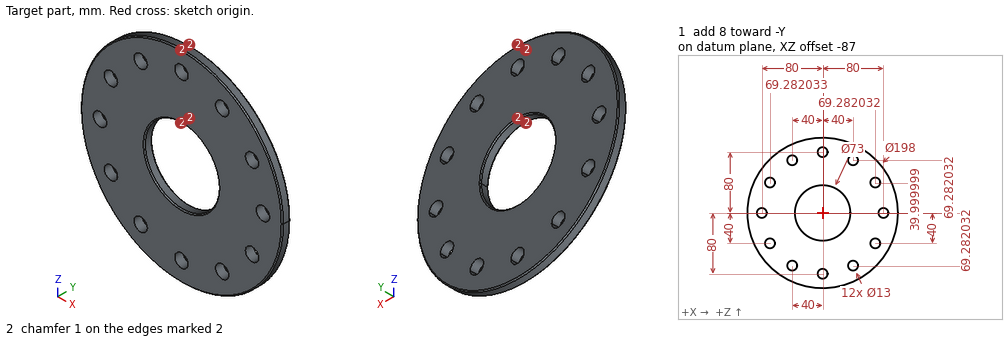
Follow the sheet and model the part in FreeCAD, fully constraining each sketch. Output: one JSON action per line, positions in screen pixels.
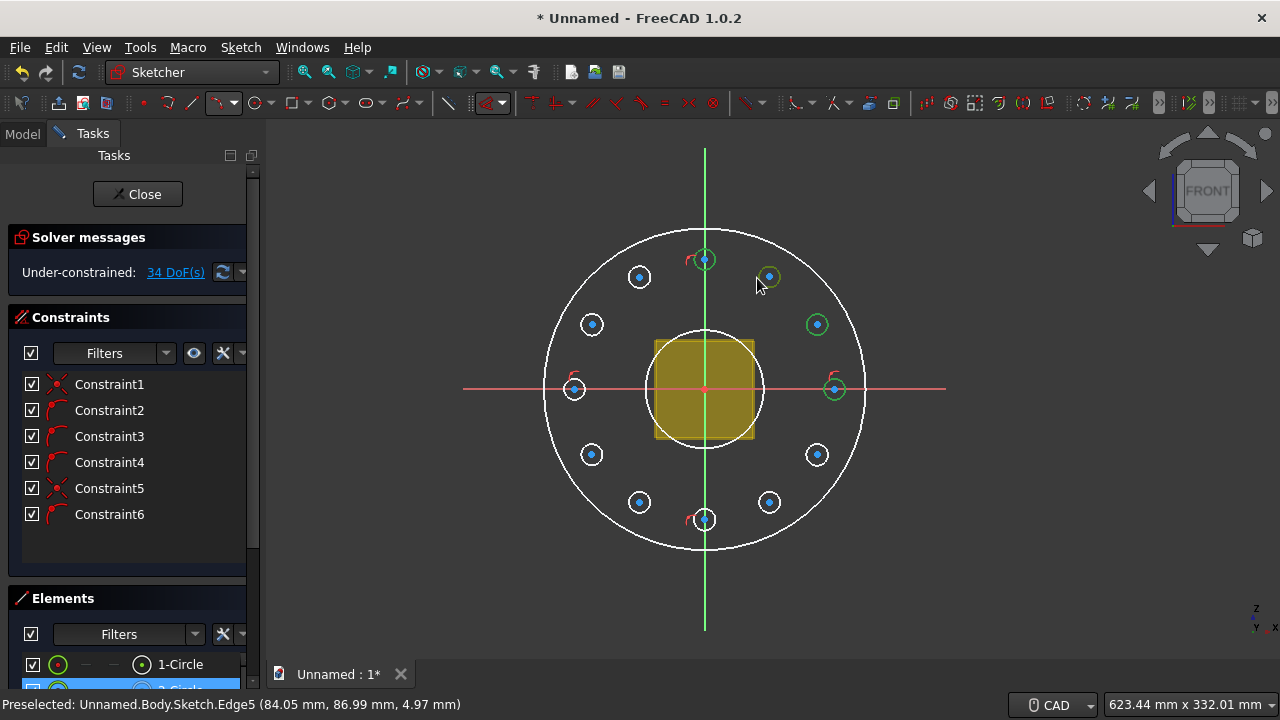
{"action": "scroll", "coordinate": [825, 447], "scroll_direction": "up", "scroll_amount": 2}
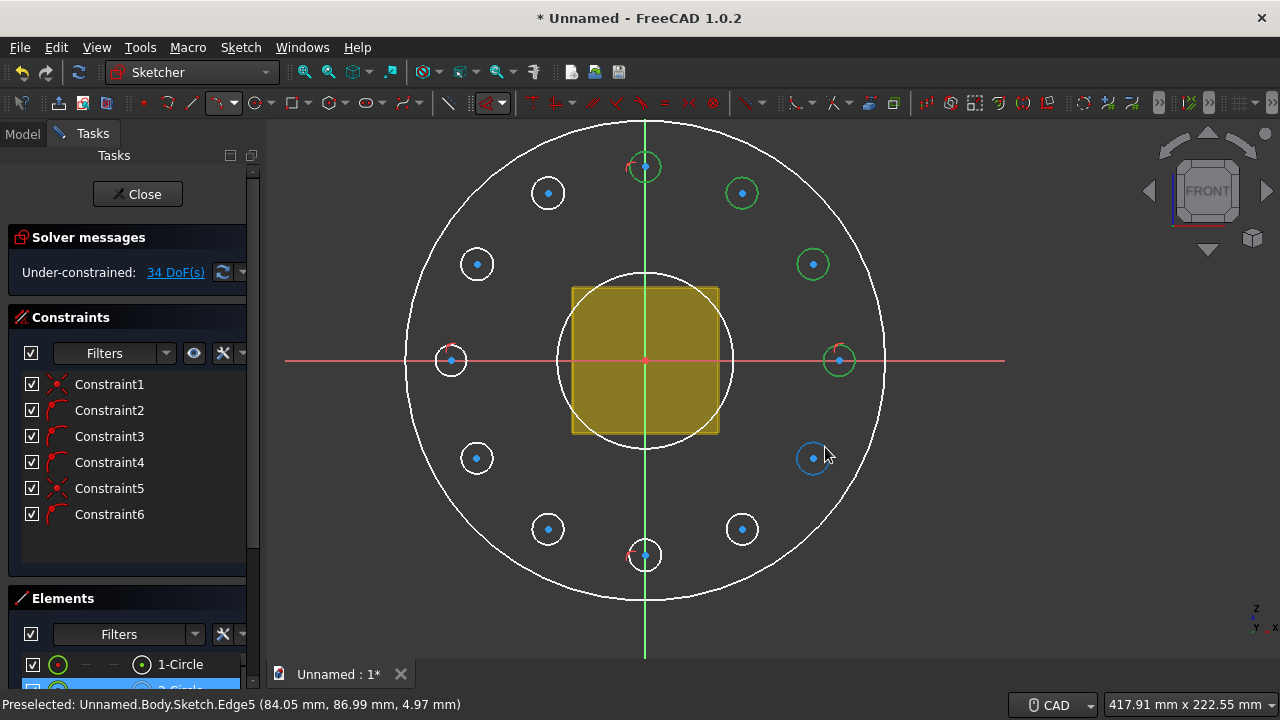
{"action": "left_click", "coordinate": [824, 447]}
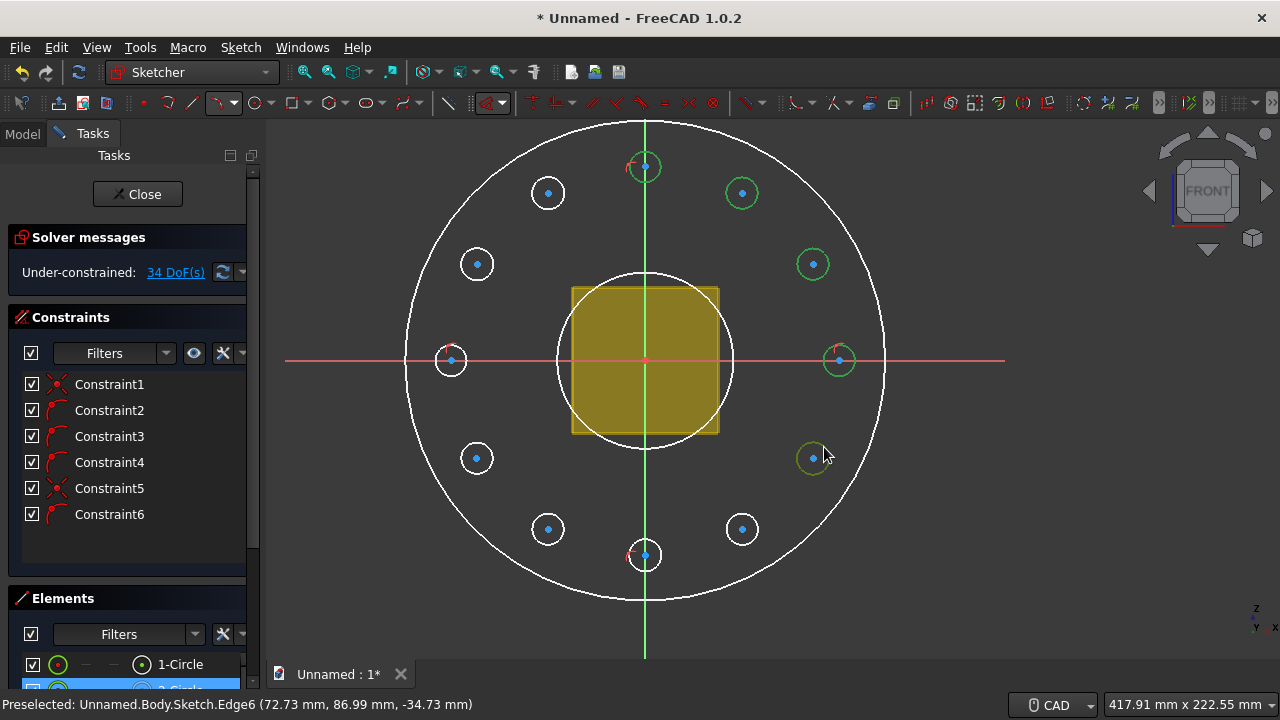
{"action": "left_click", "coordinate": [753, 518]}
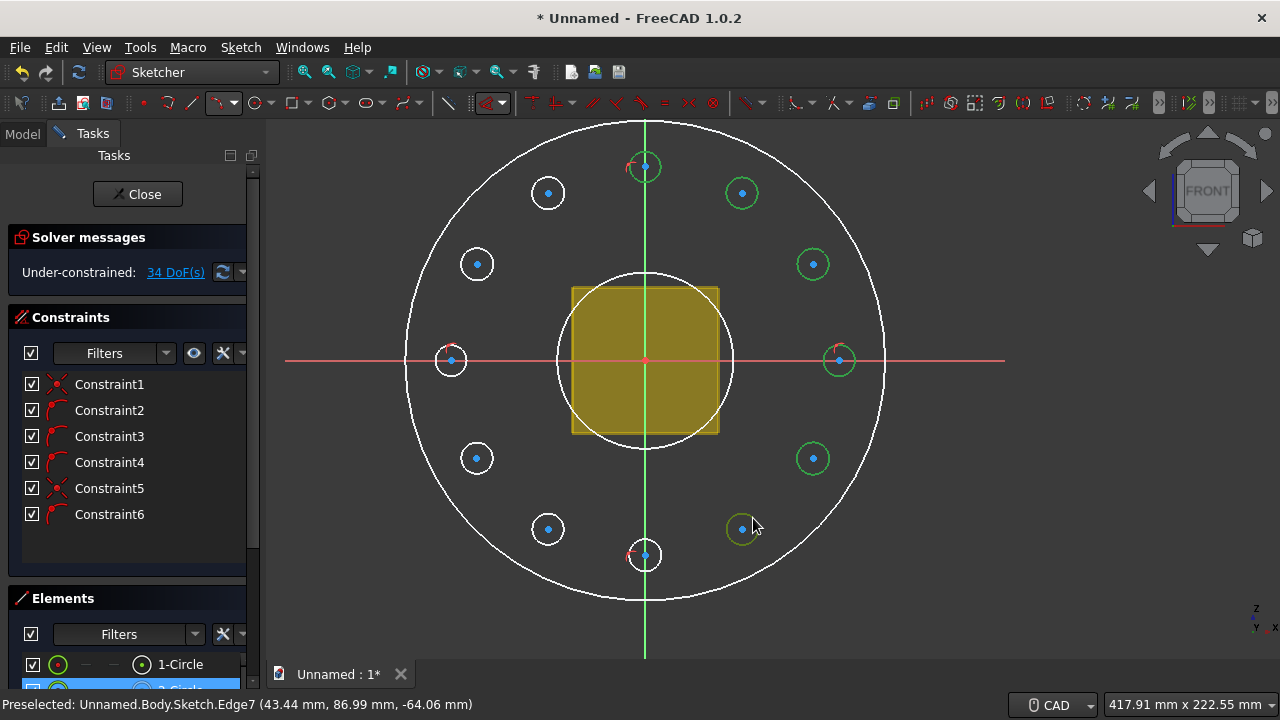
{"action": "left_click", "coordinate": [560, 182]}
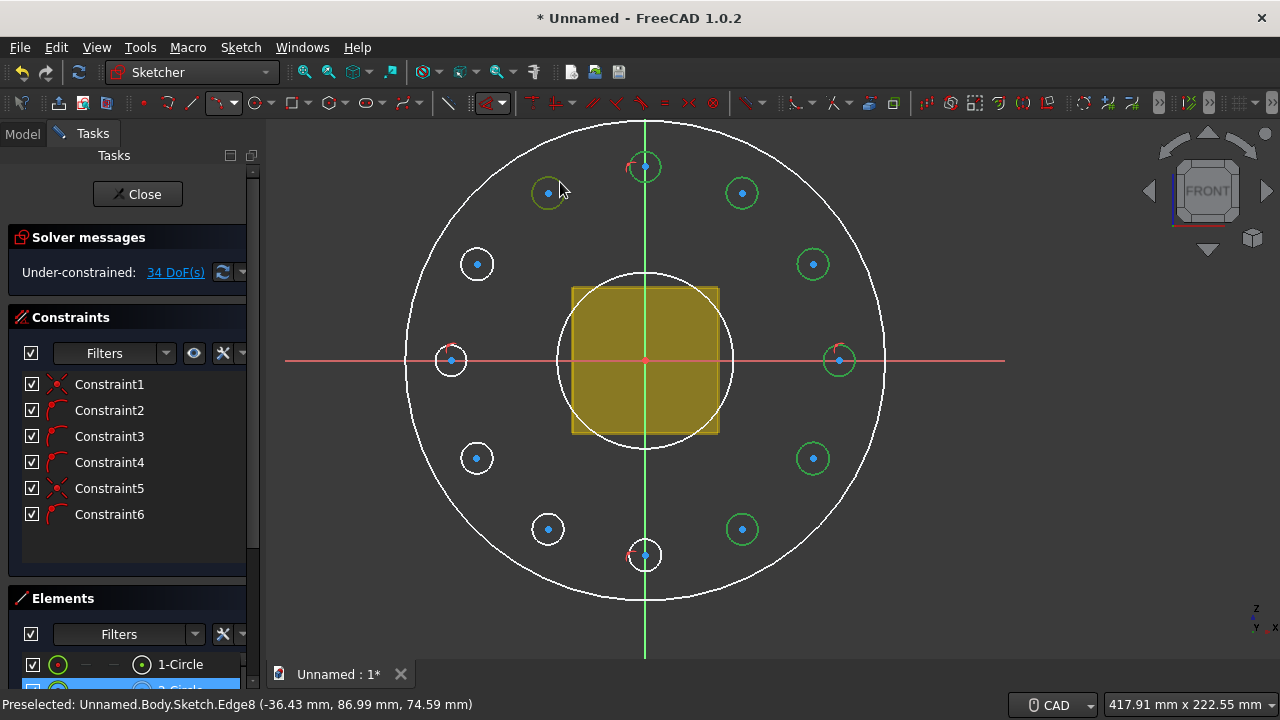
{"action": "left_click", "coordinate": [489, 253]}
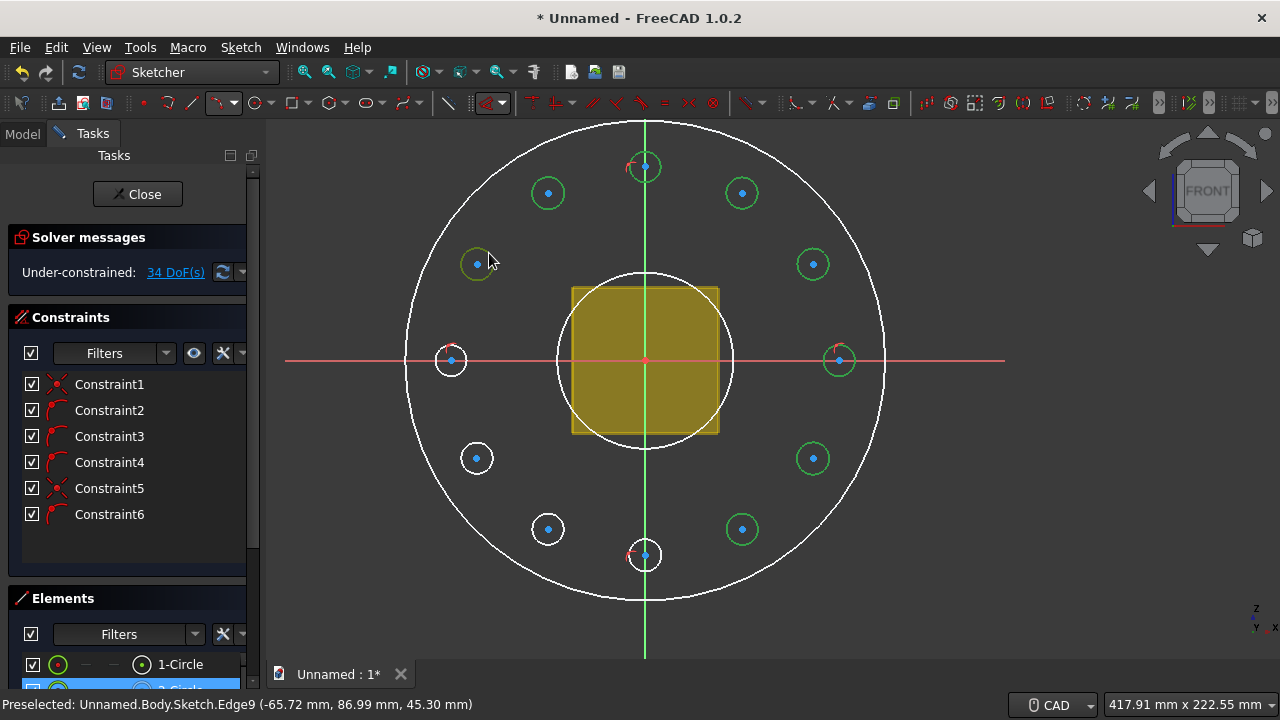
{"action": "scroll", "coordinate": [462, 350], "scroll_direction": "up", "scroll_amount": 2}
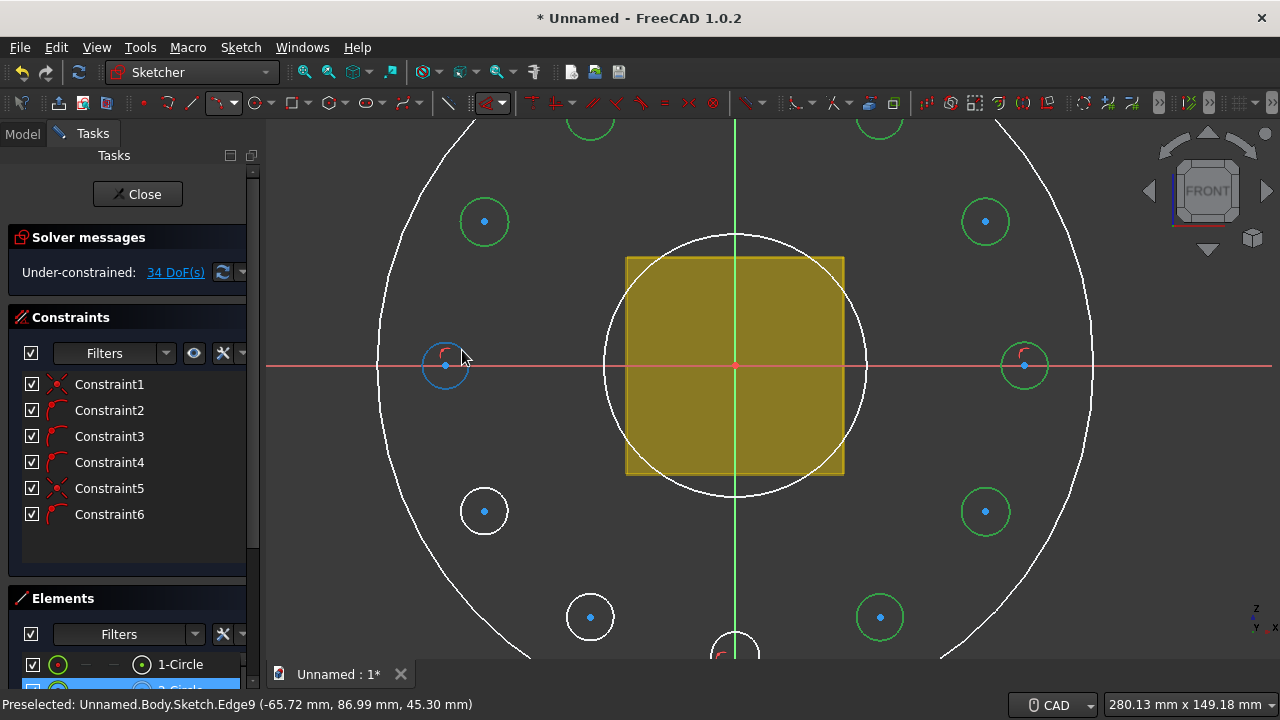
{"action": "left_click", "coordinate": [462, 349]}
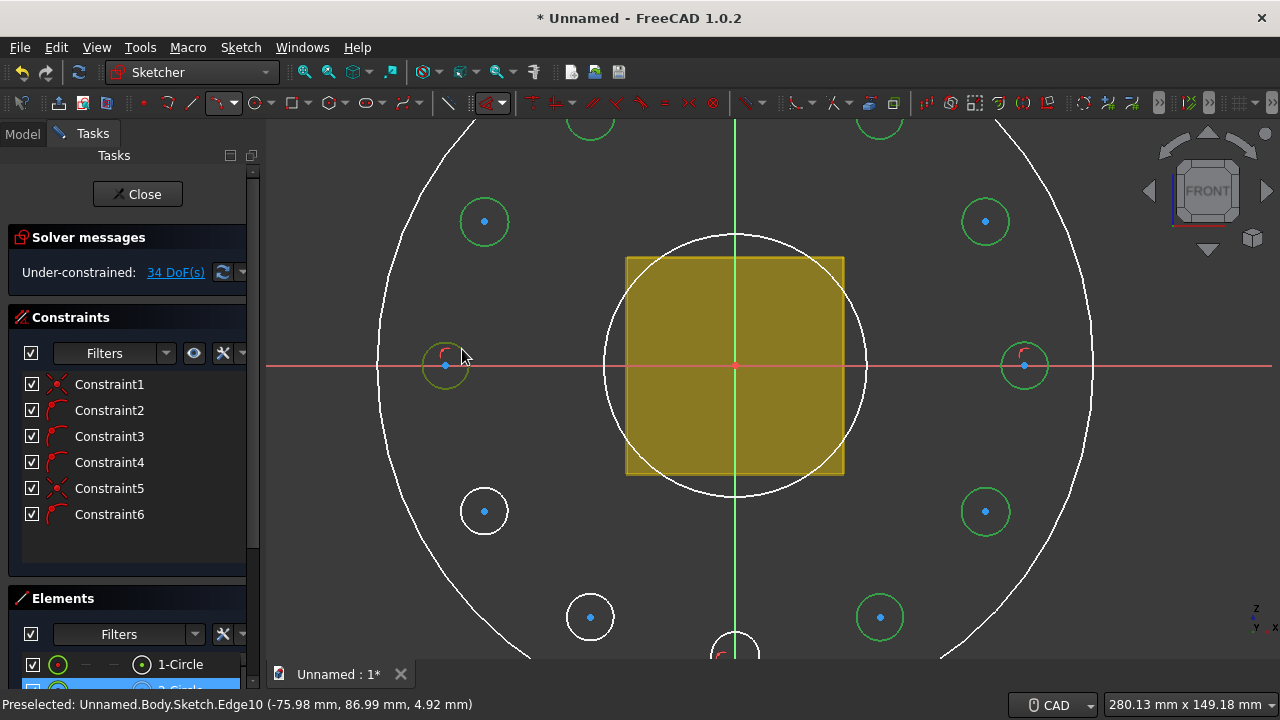
{"action": "scroll", "coordinate": [679, 408], "scroll_direction": "down", "scroll_amount": 4}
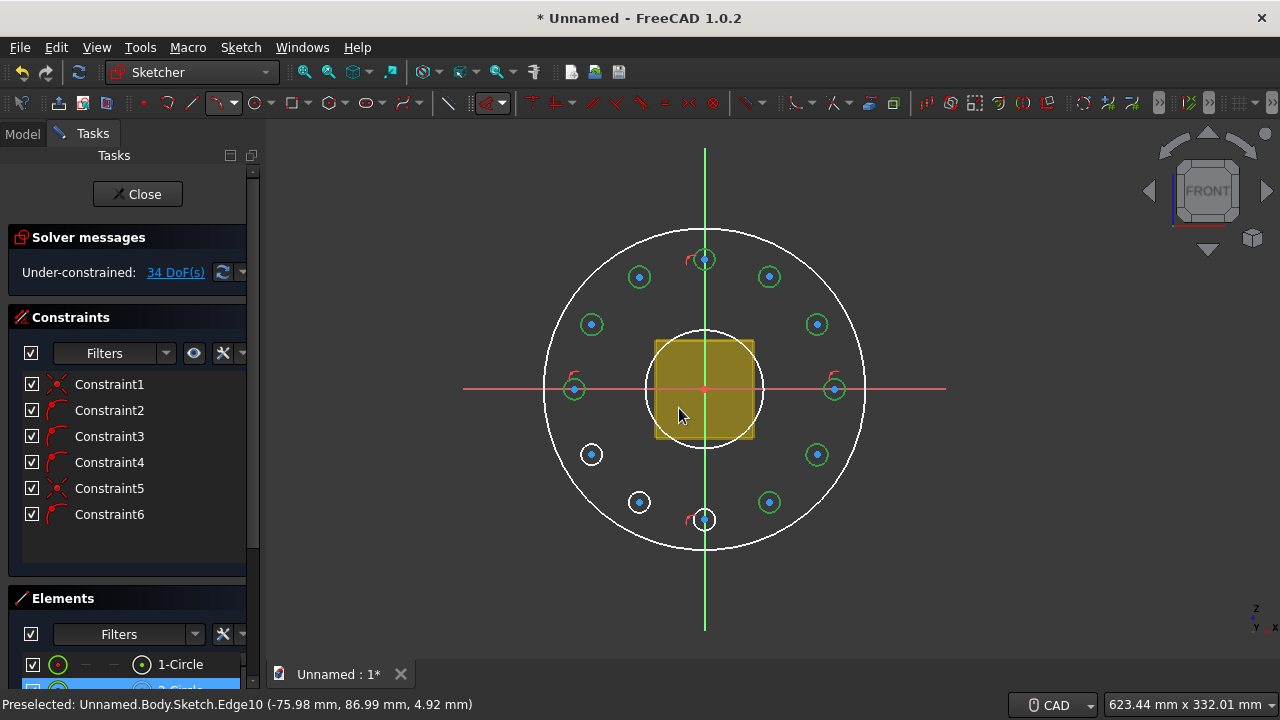
{"action": "scroll", "coordinate": [712, 512], "scroll_direction": "up", "scroll_amount": 3}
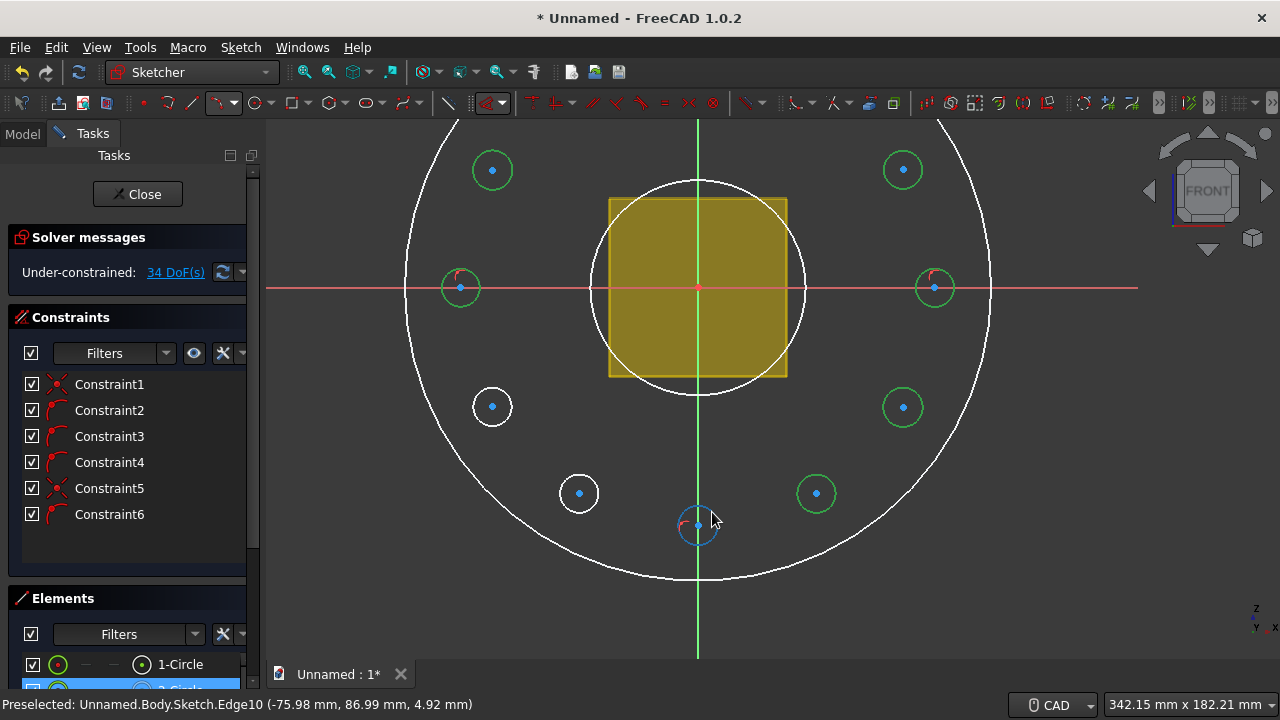
{"action": "left_click", "coordinate": [712, 512]}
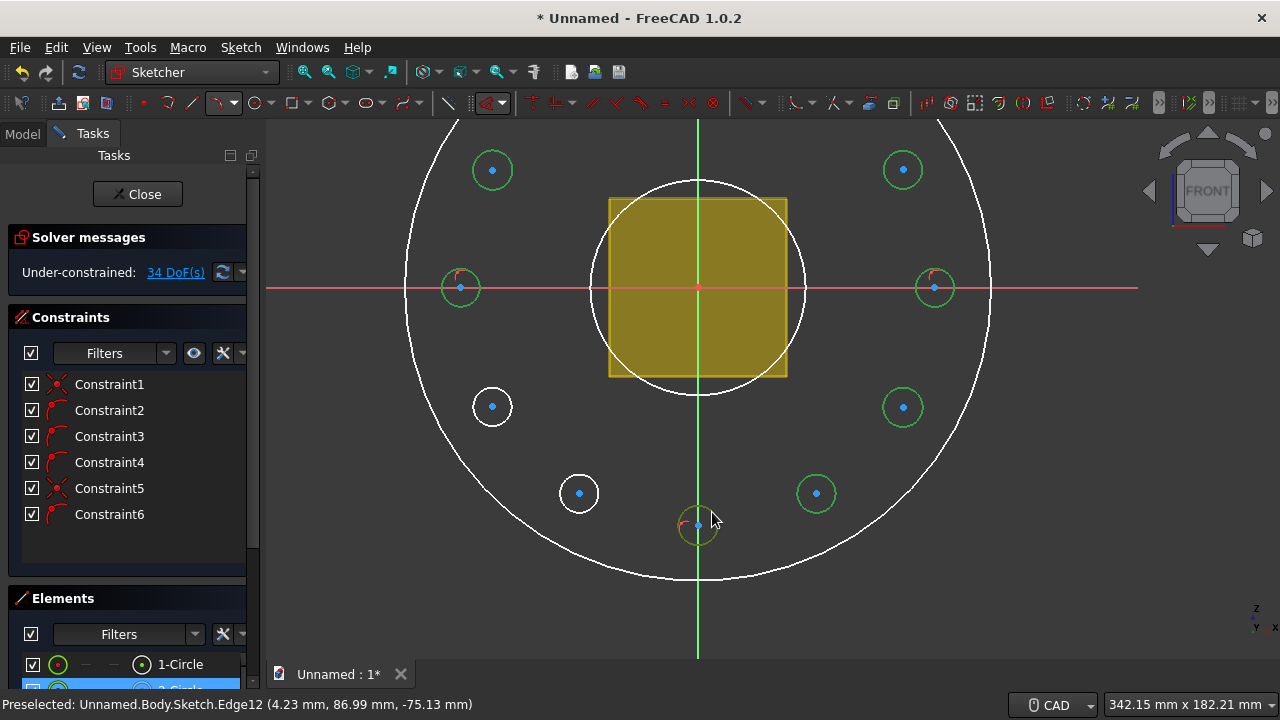
{"action": "left_click", "coordinate": [593, 480]}